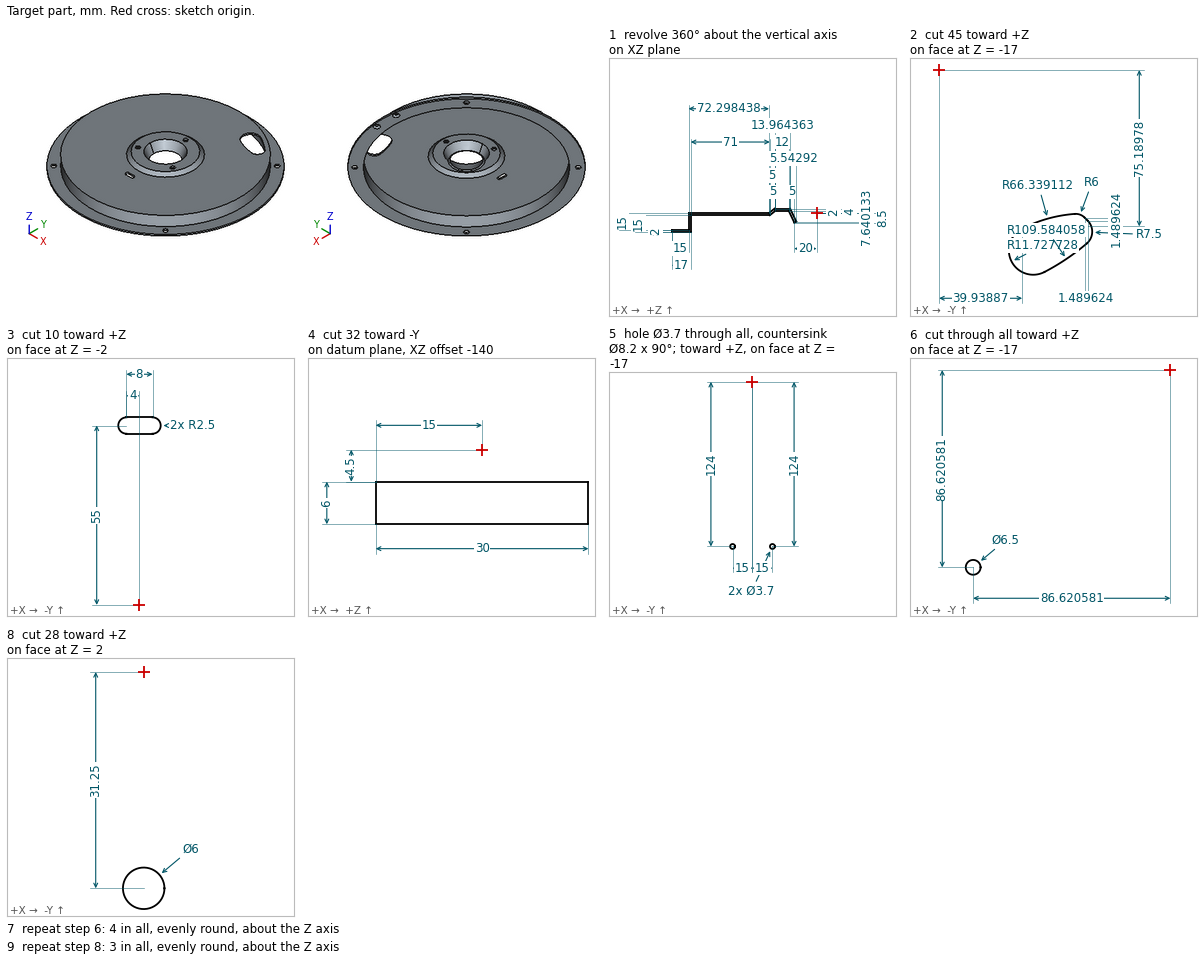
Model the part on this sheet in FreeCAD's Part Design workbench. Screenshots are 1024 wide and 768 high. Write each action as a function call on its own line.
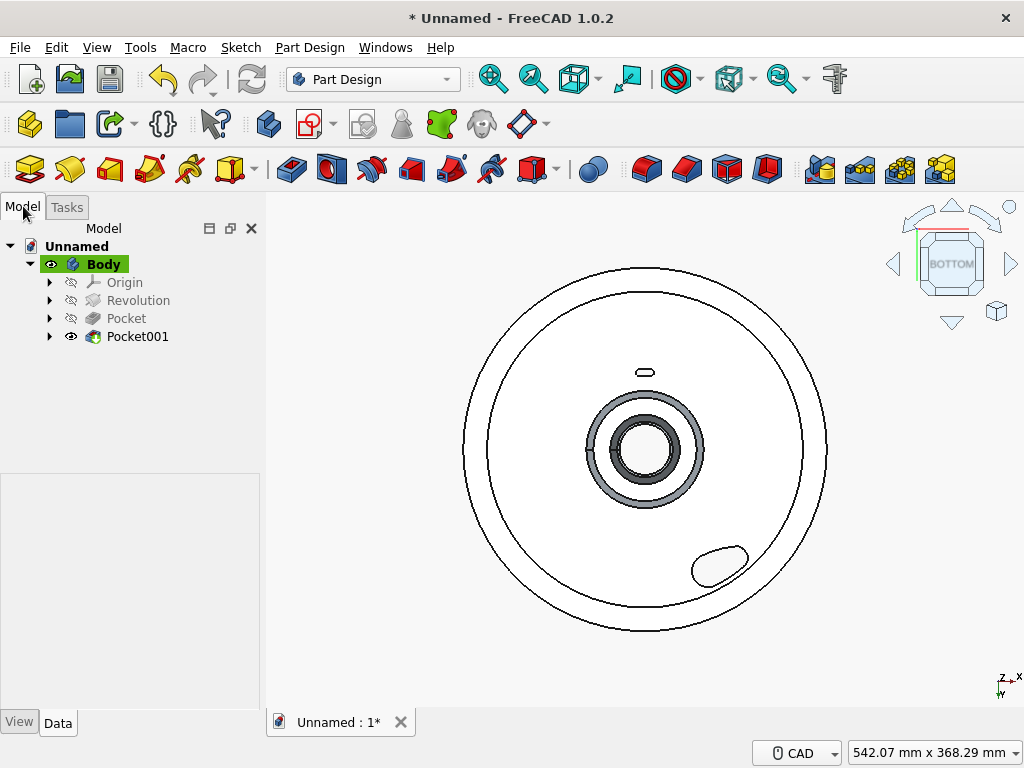
click(50, 282)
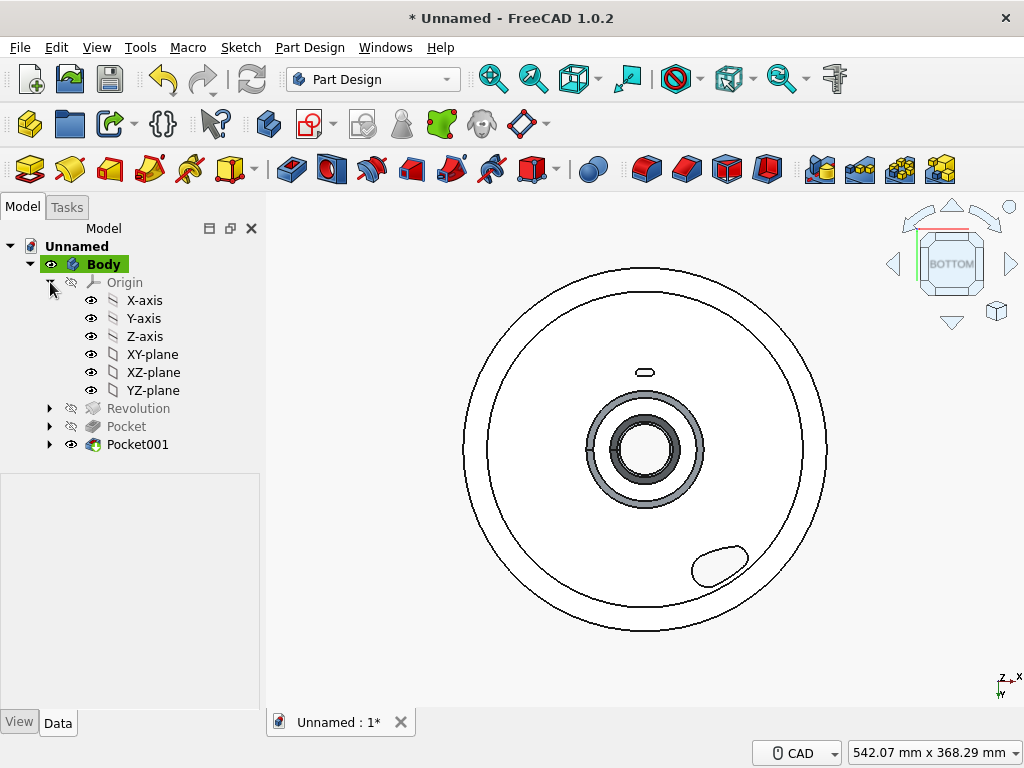
click(136, 372)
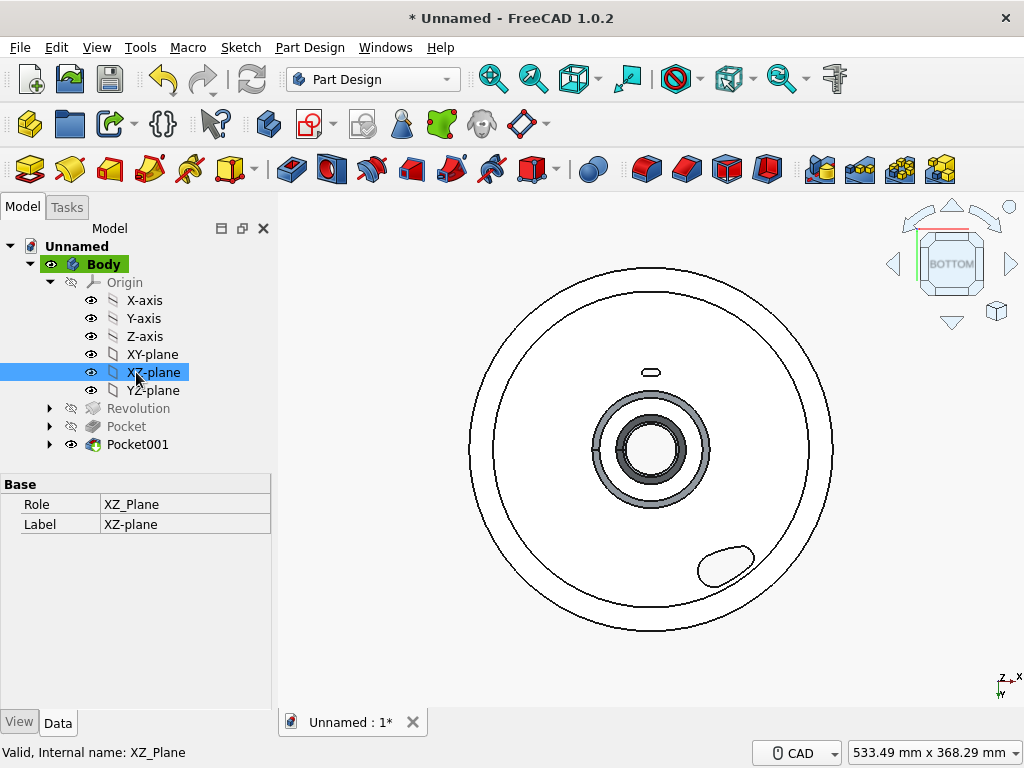
click(522, 124)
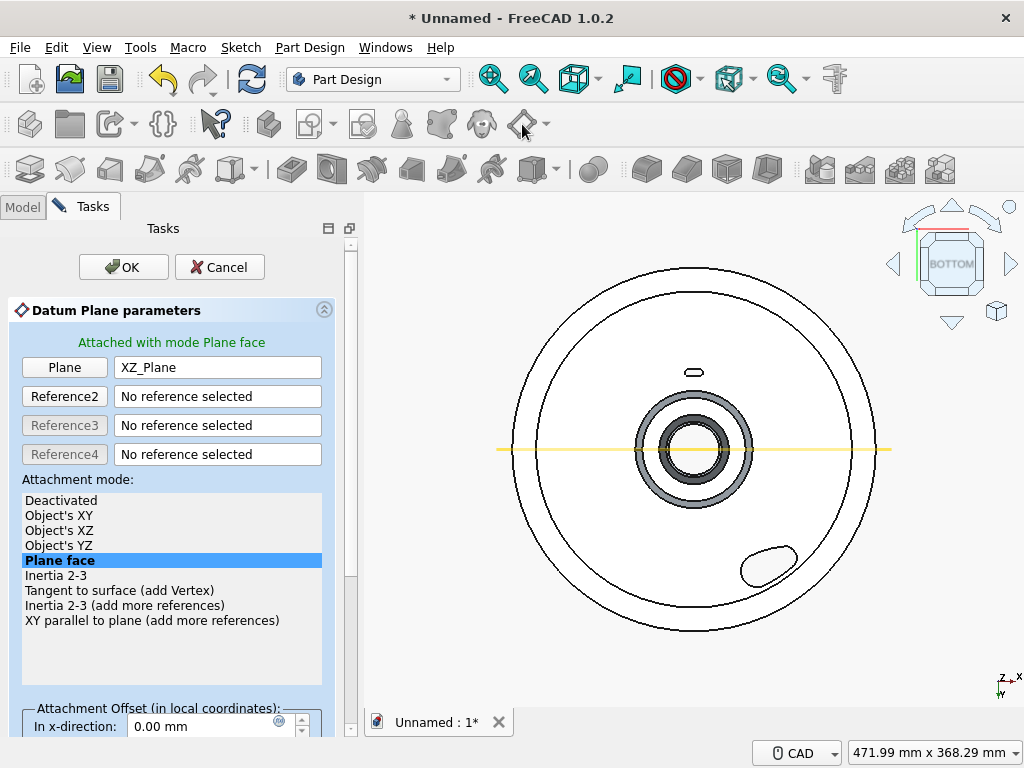
scroll(351, 487, down, 3)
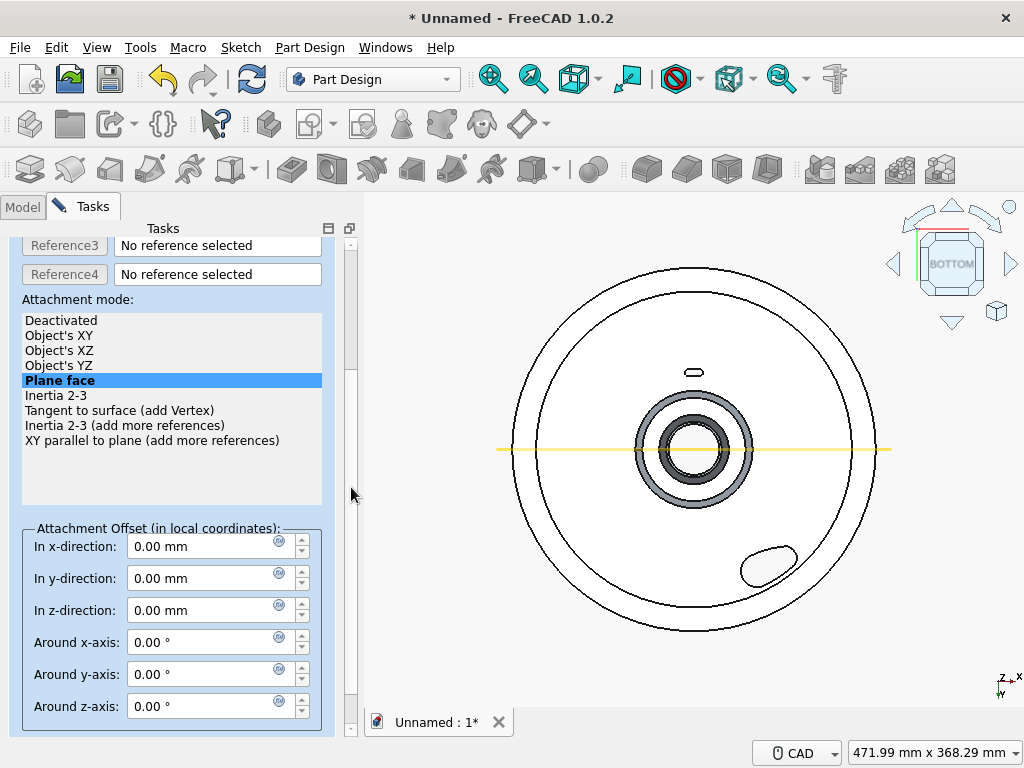
triple_click(210, 610)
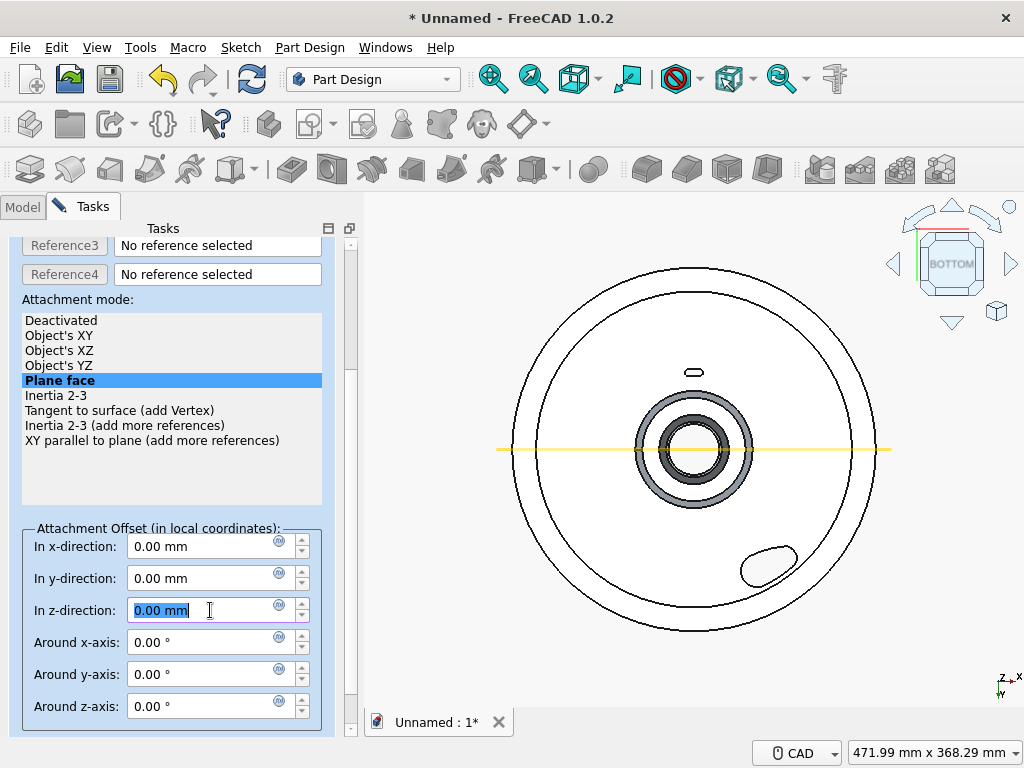
text(-140)
key(Tab)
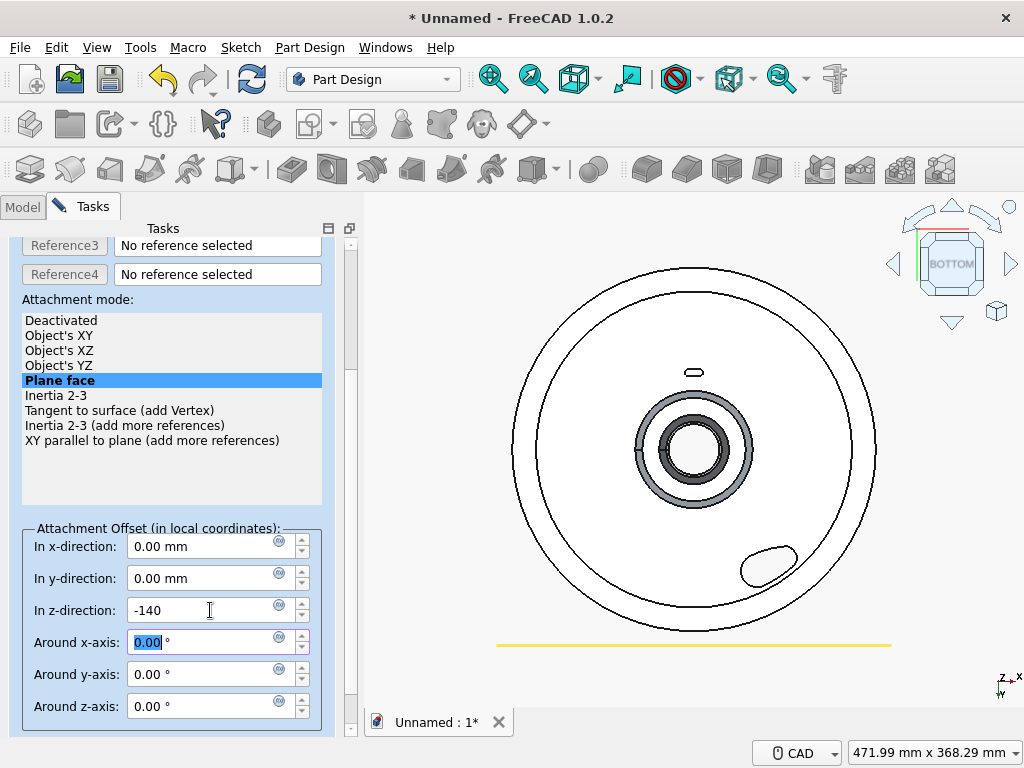
scroll(351, 487, up, 4)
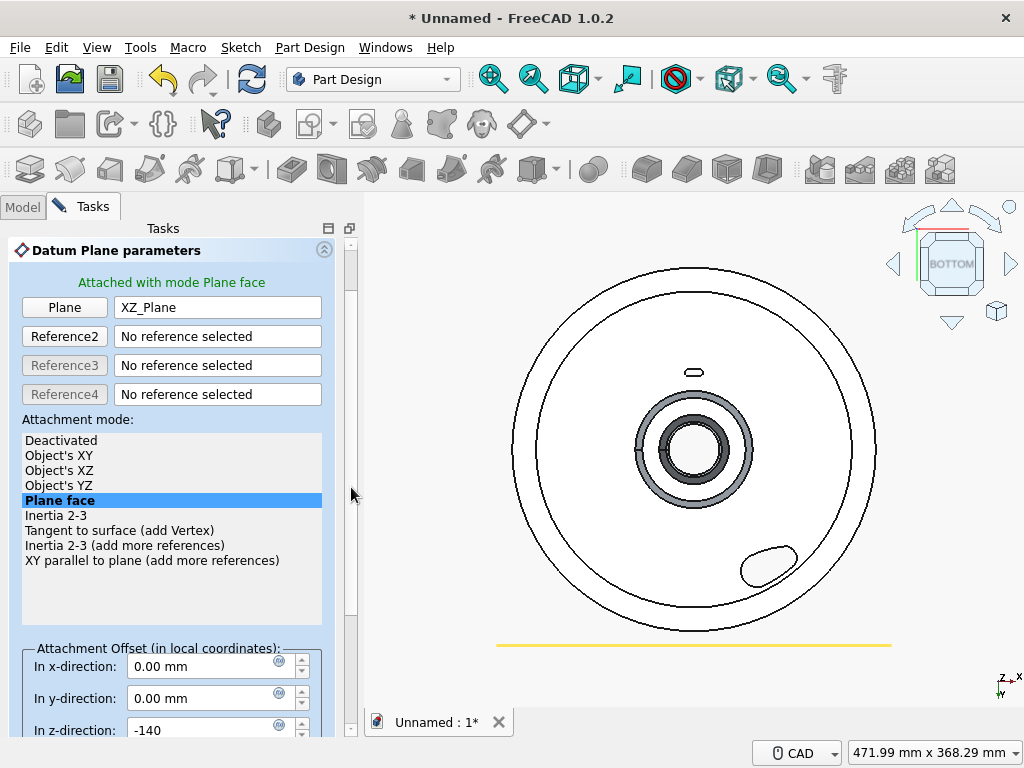
click(124, 267)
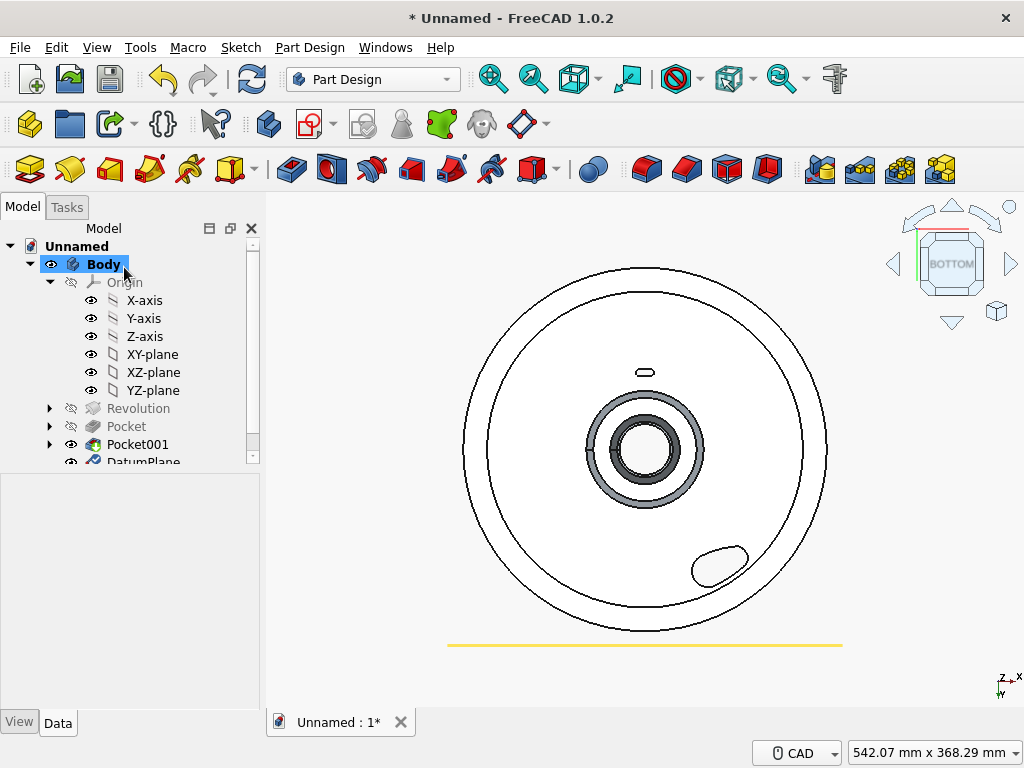
click(116, 462)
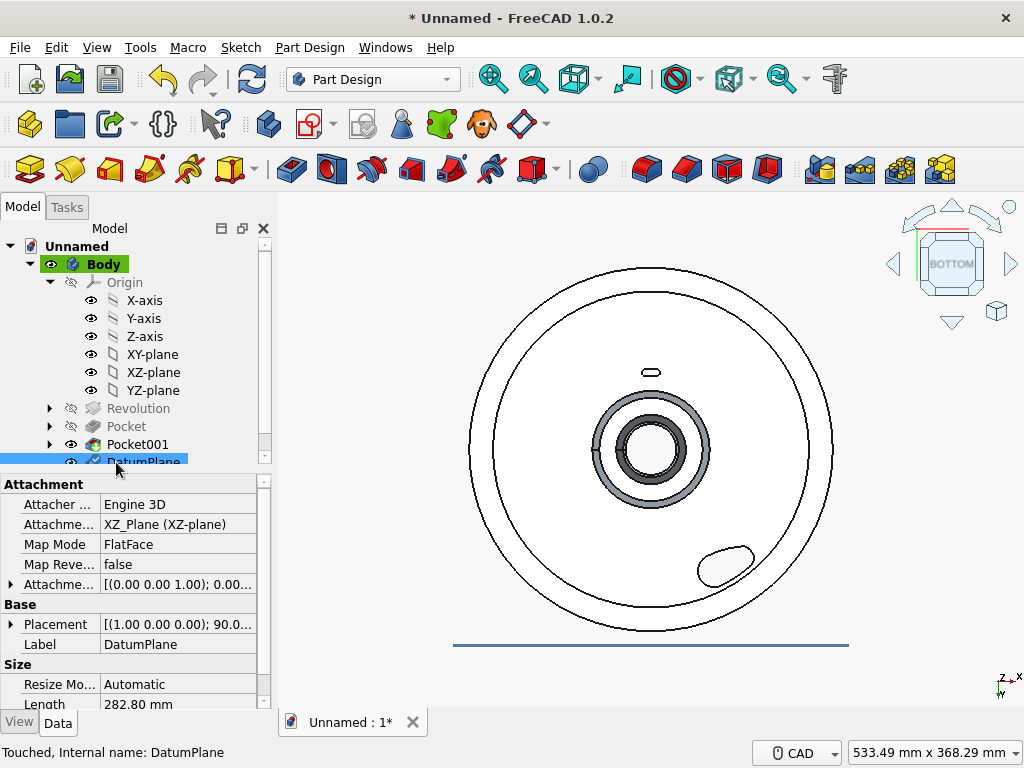
click(310, 124)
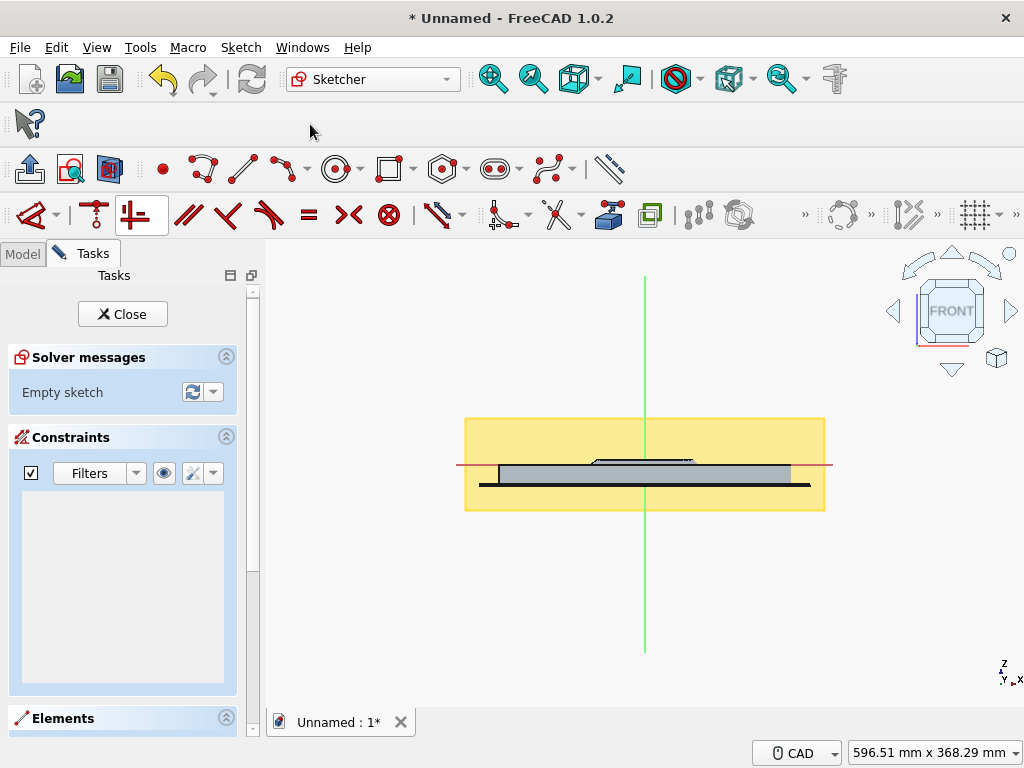
click(110, 170)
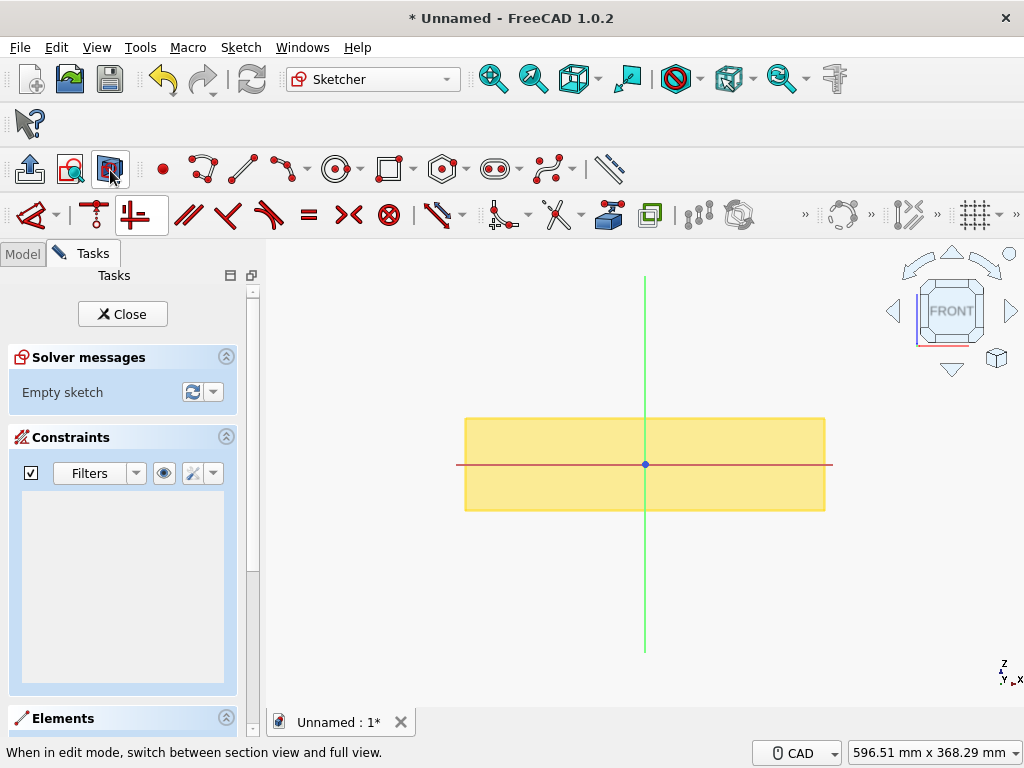
scroll(652, 471, up, 12)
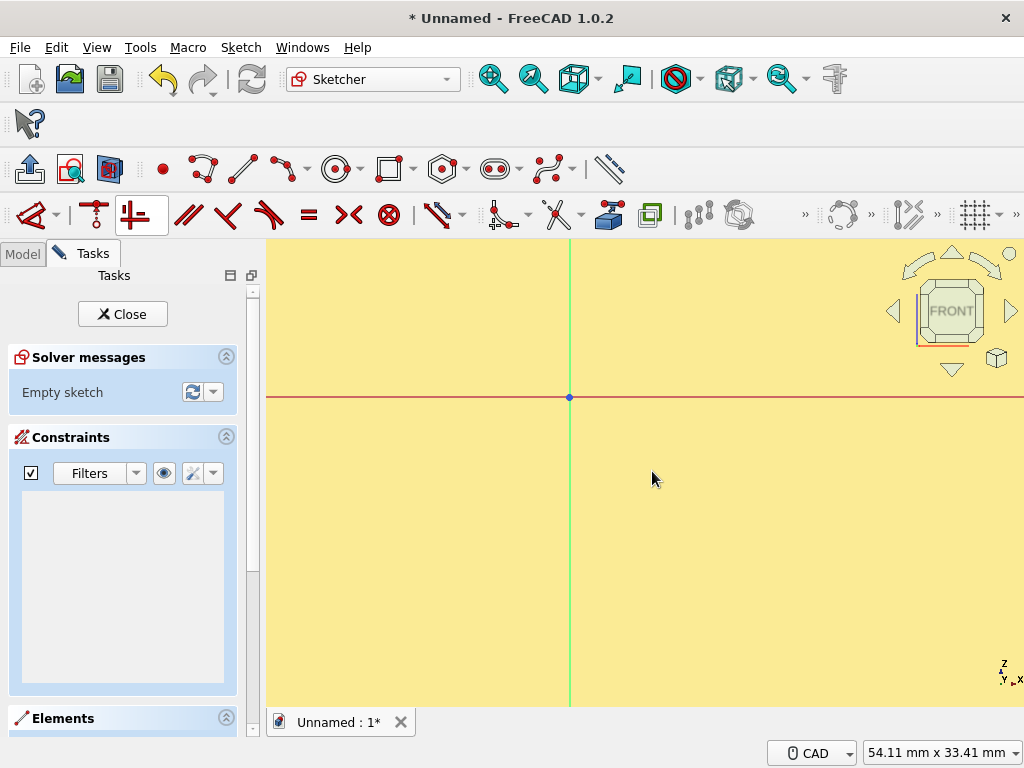
key(g)
key(r)